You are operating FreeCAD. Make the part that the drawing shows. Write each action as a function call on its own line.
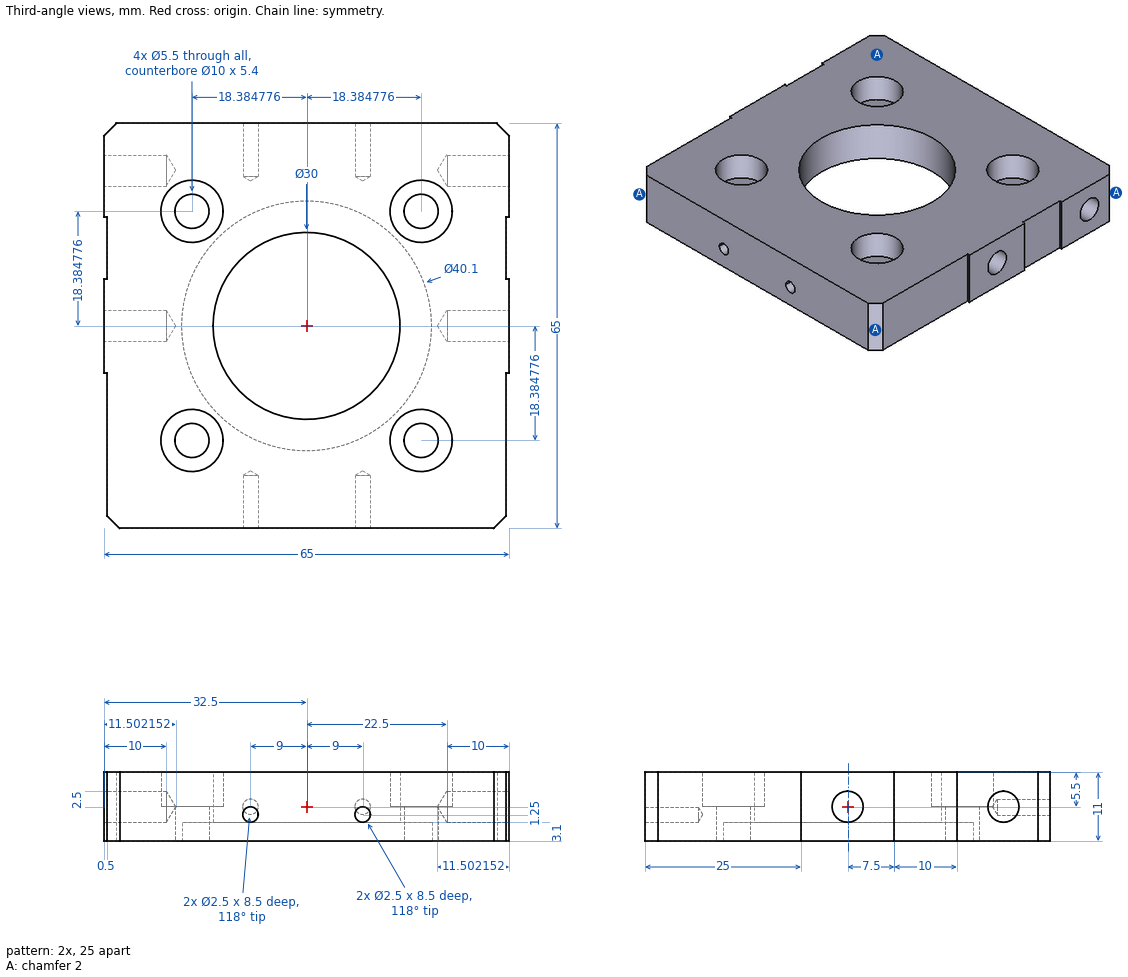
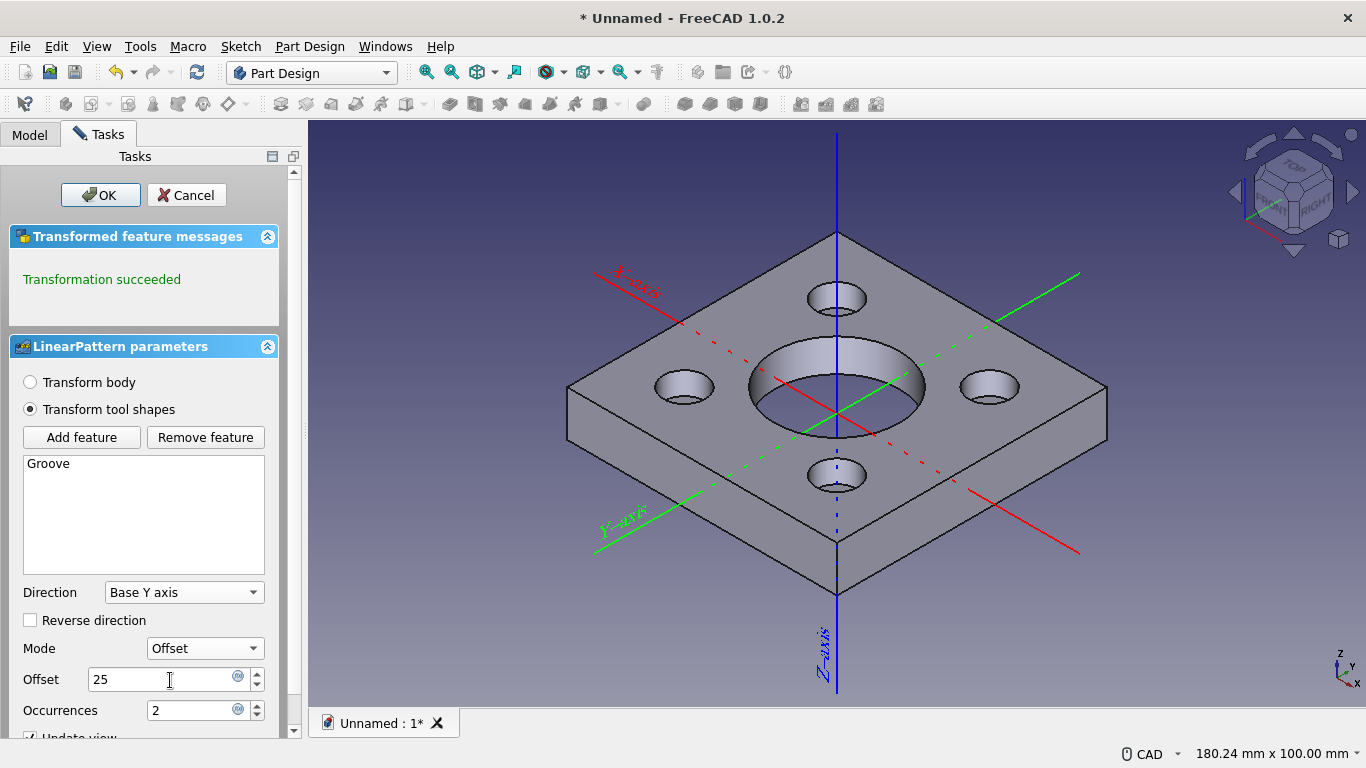
triple_click(199, 710)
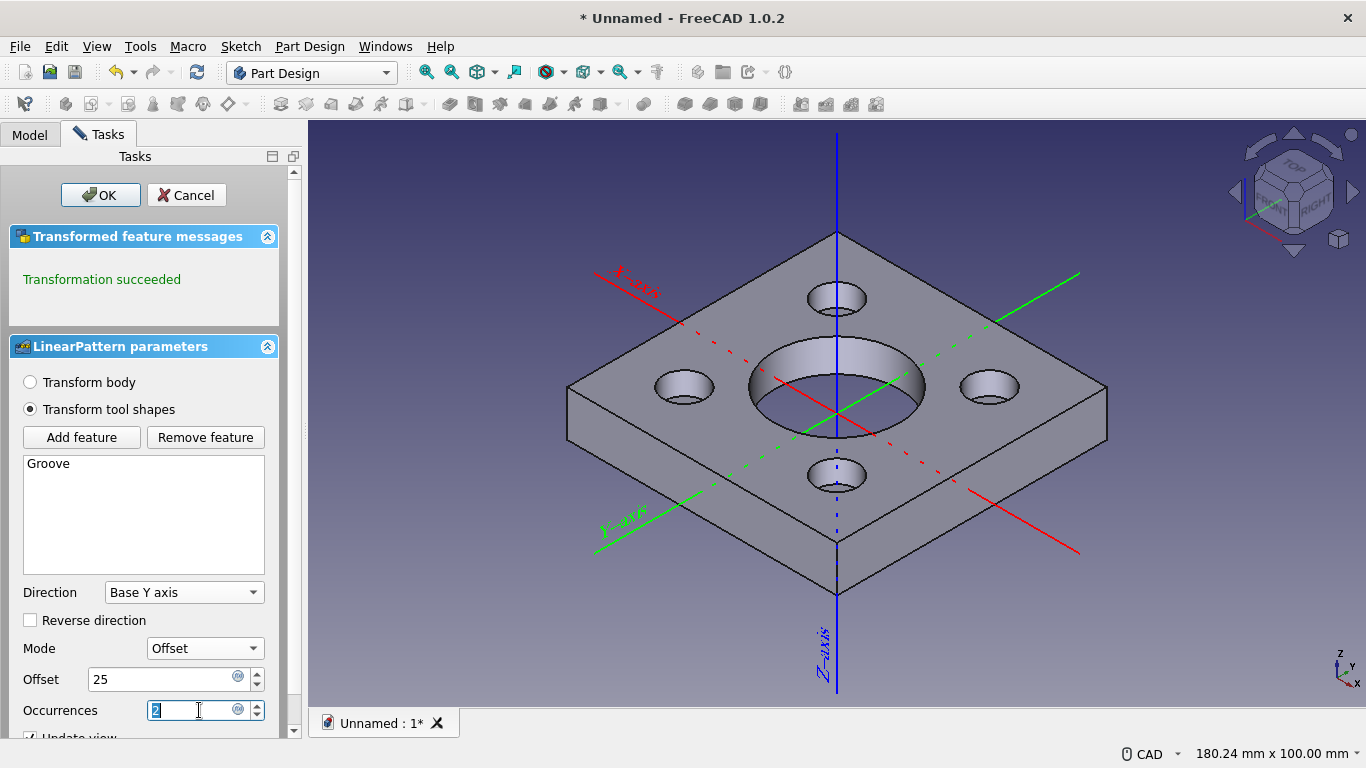
text(2)
key(Tab)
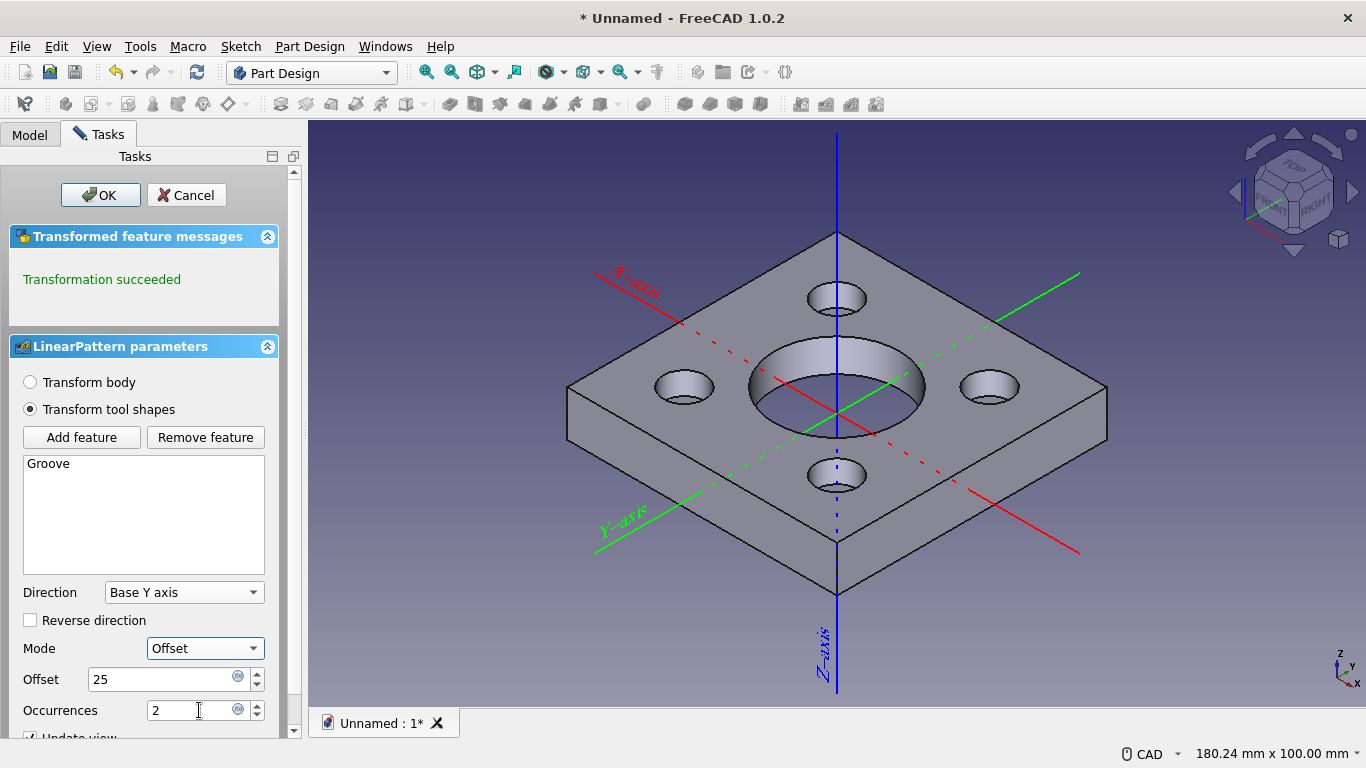
click(101, 195)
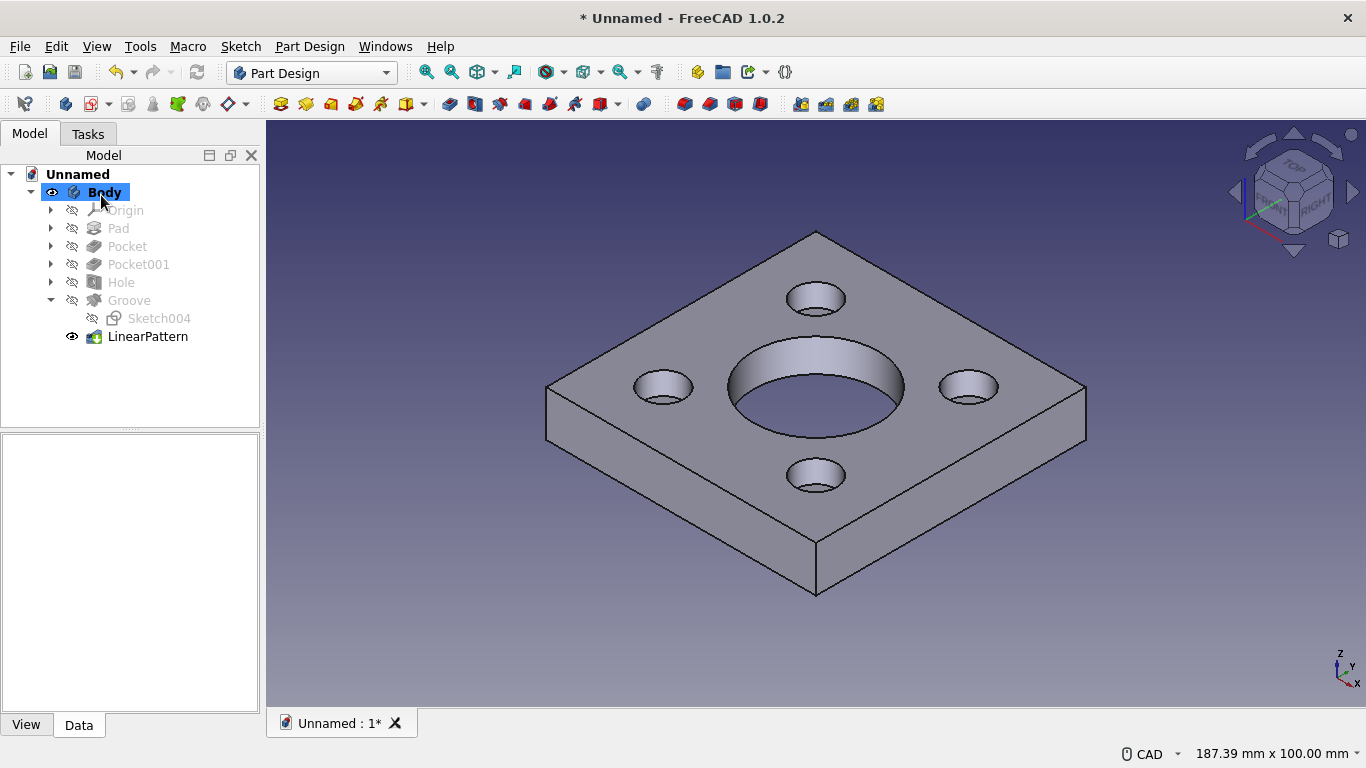
key(6)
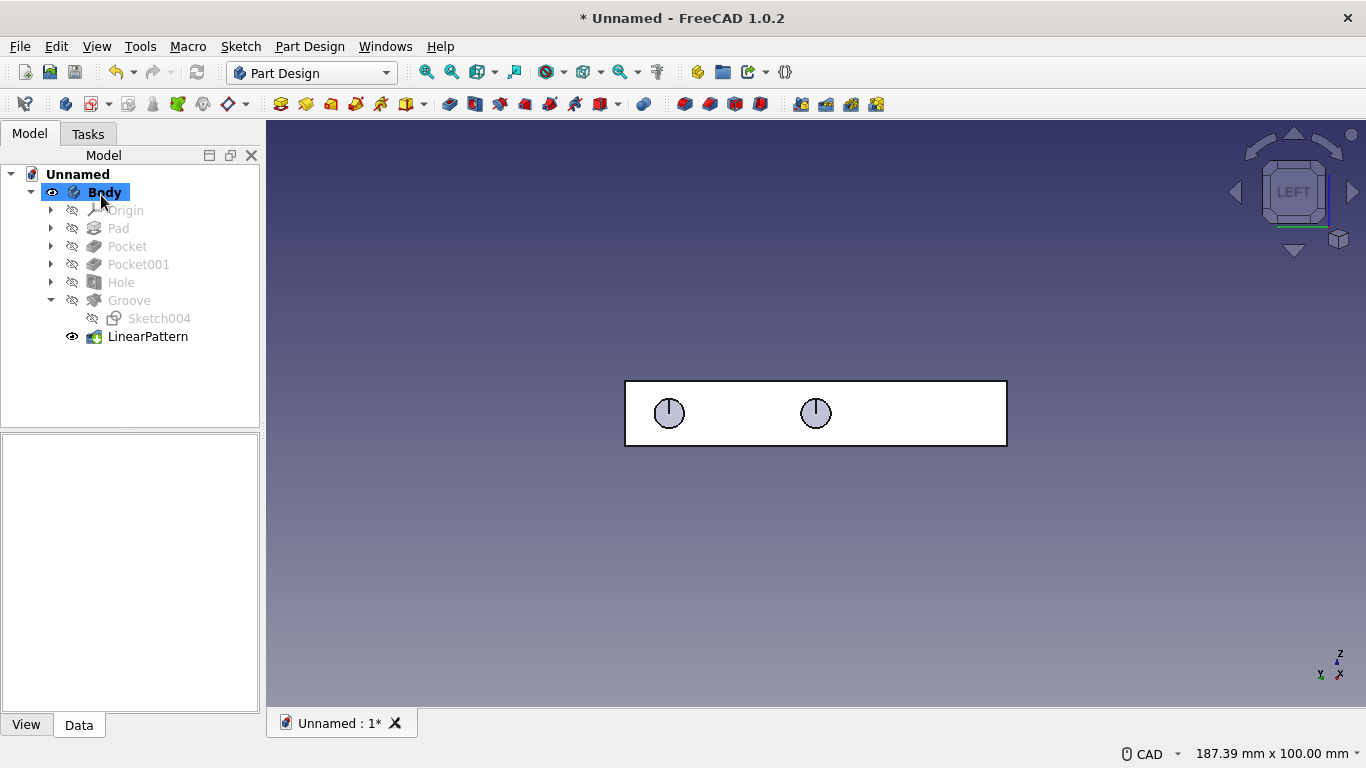
click(427, 72)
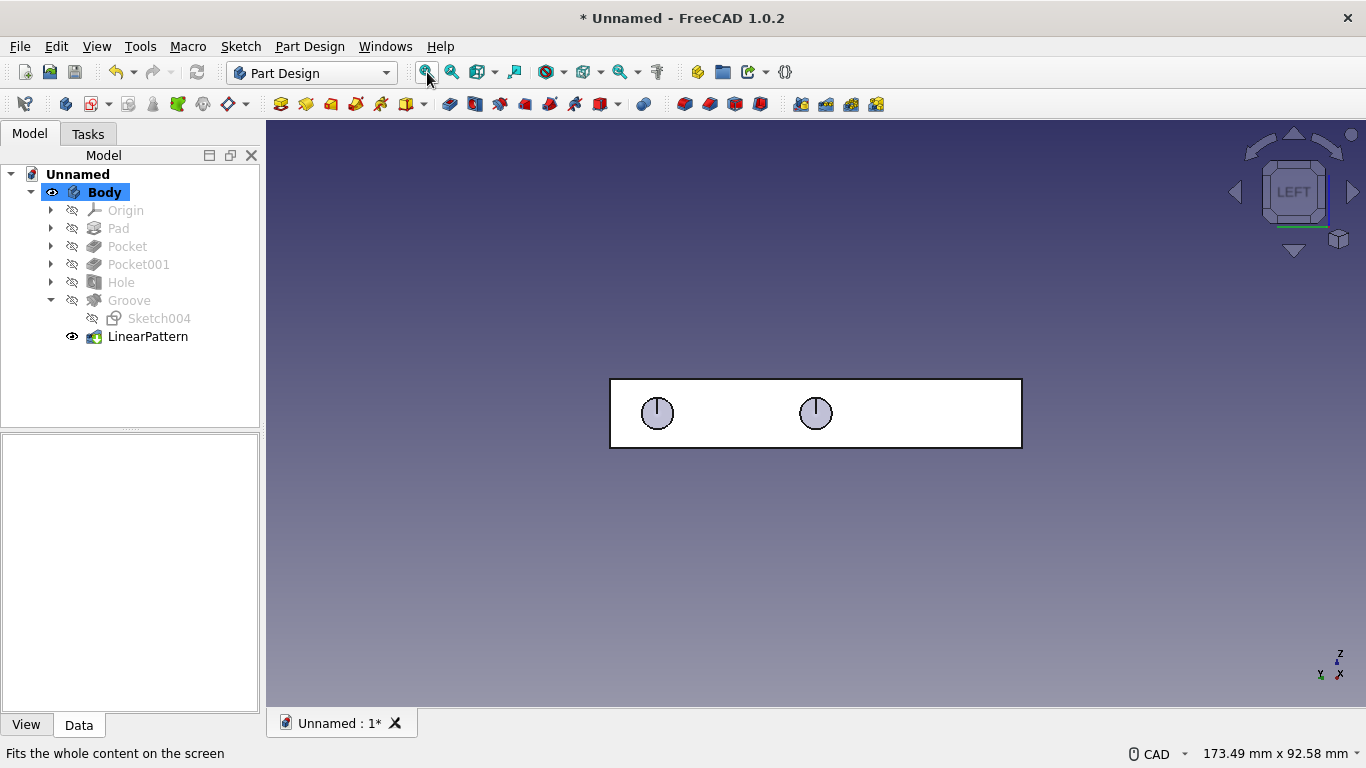
click(757, 412)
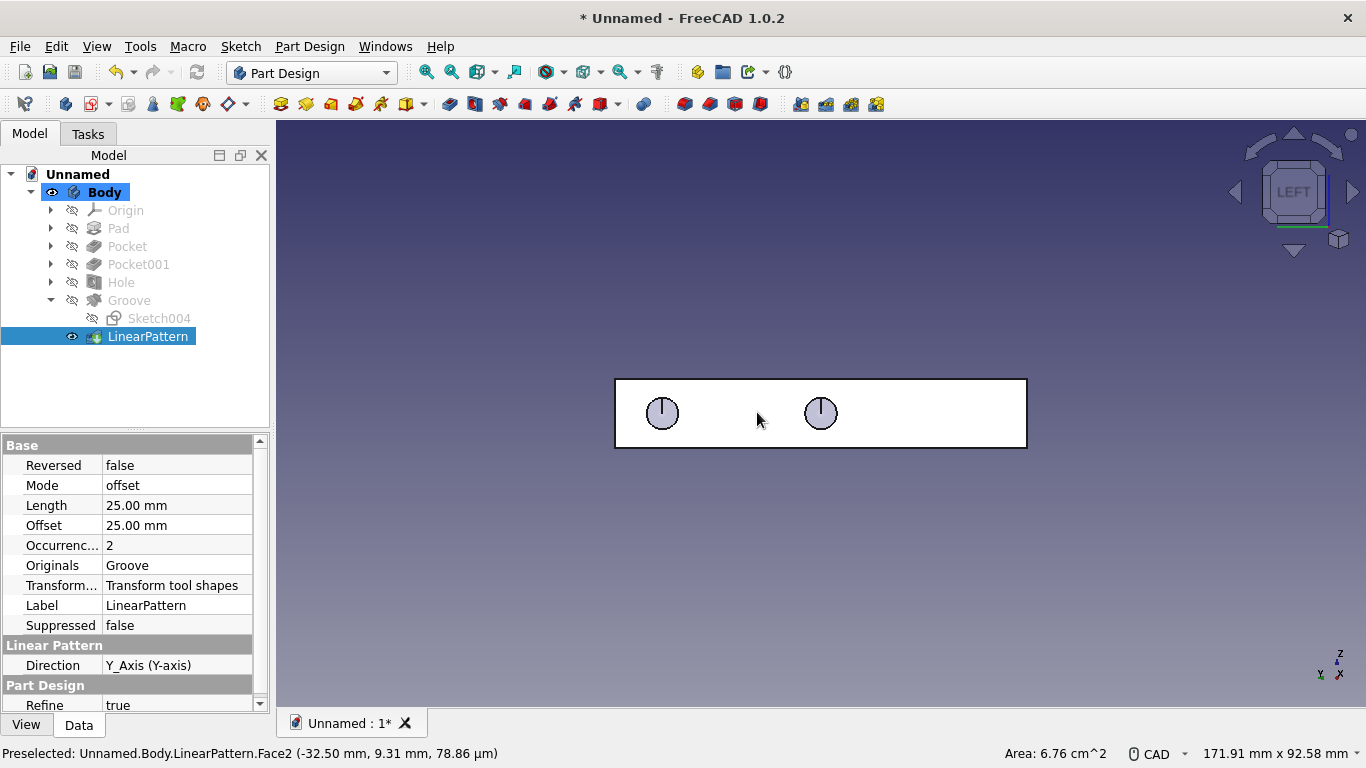
click(90, 104)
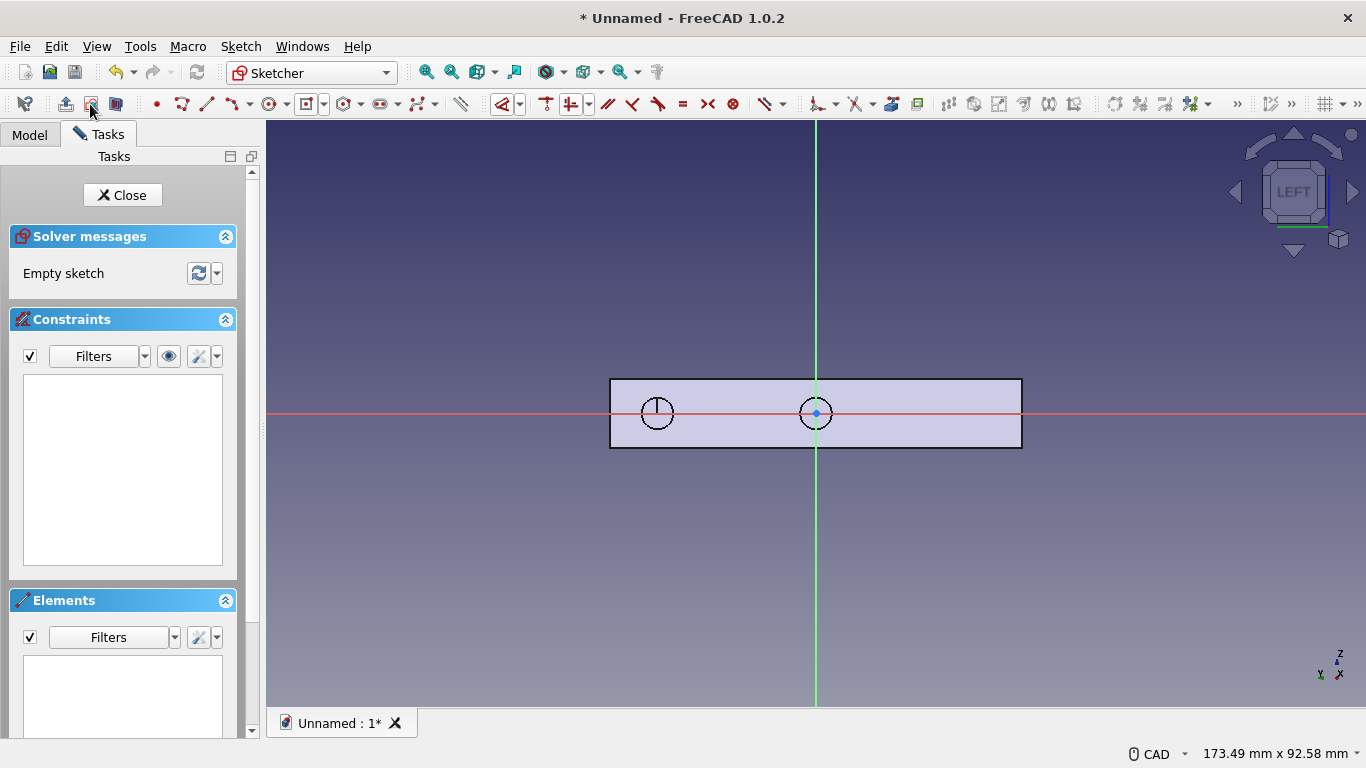
scroll(958, 413, up, 4)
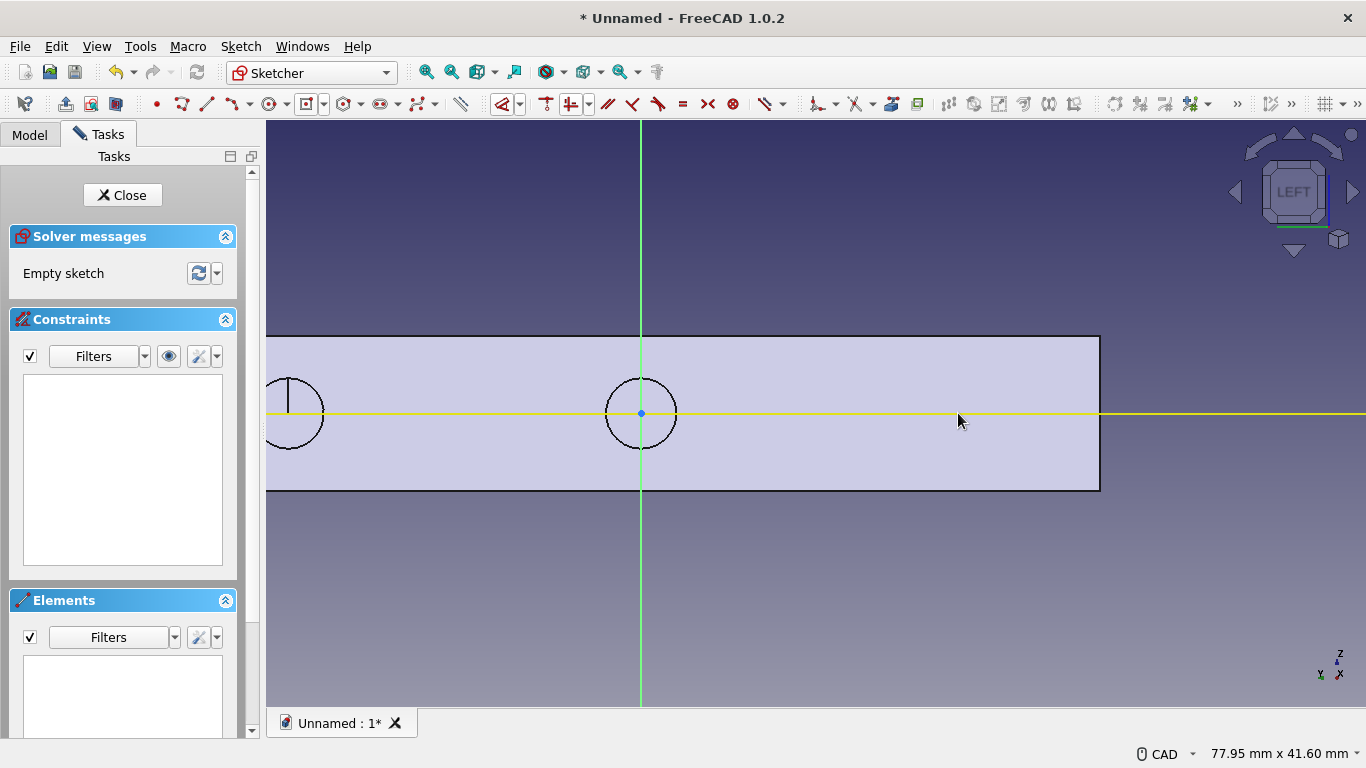
click(324, 104)